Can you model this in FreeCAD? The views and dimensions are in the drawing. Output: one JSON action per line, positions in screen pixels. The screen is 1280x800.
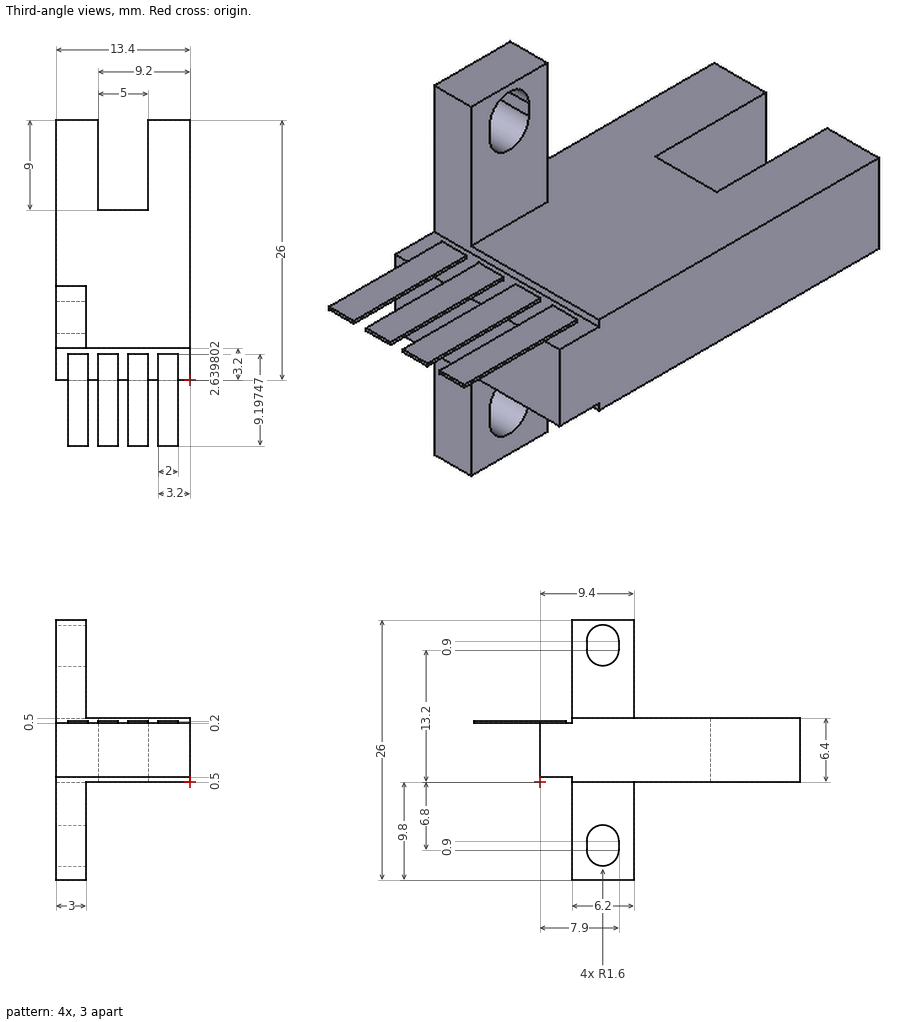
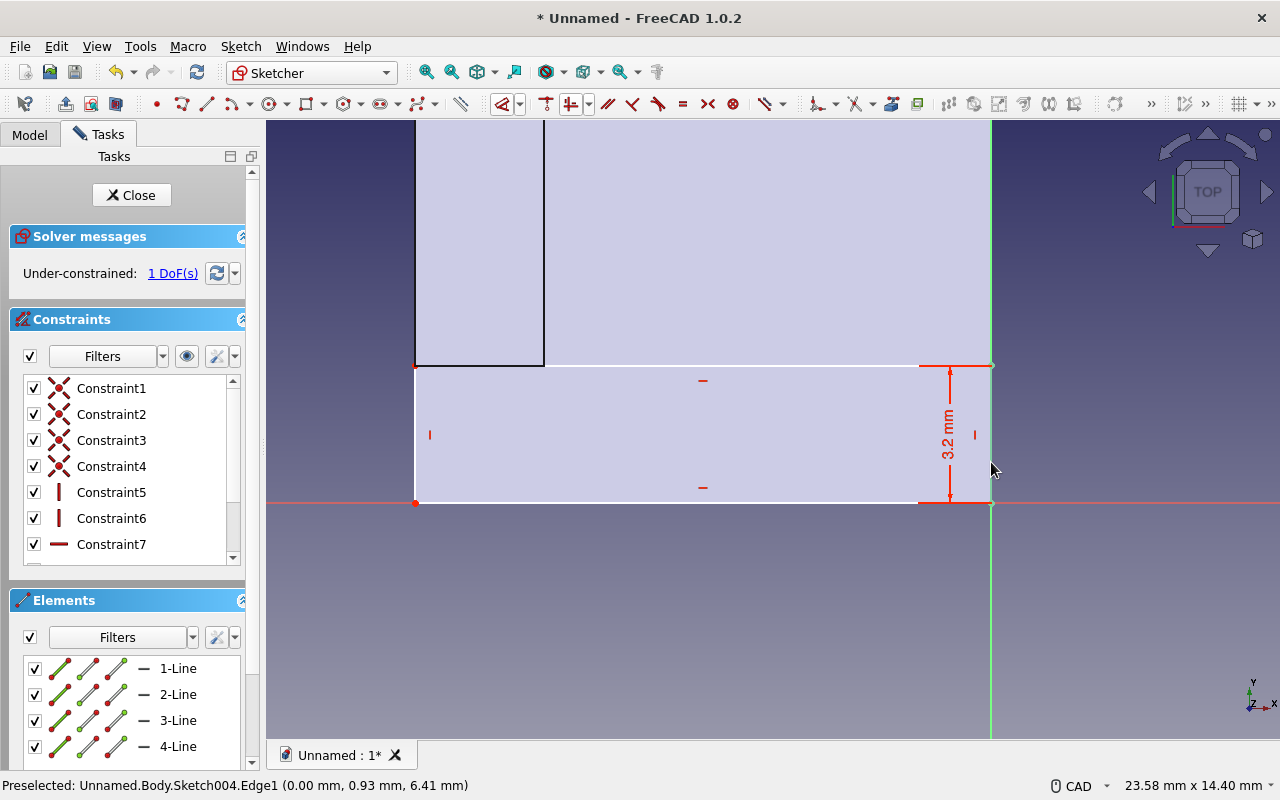
{"action": "left_click", "coordinate": [818, 366]}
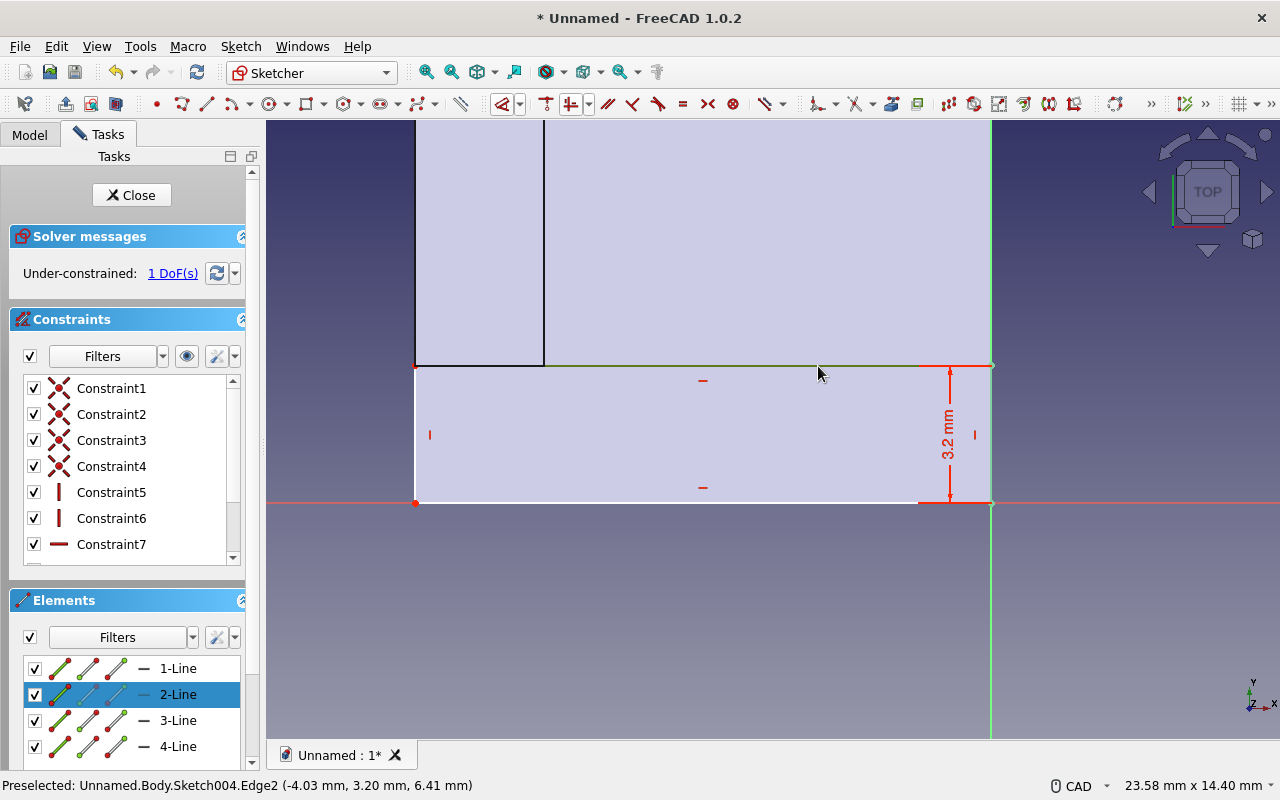
{"action": "key", "text": "l"}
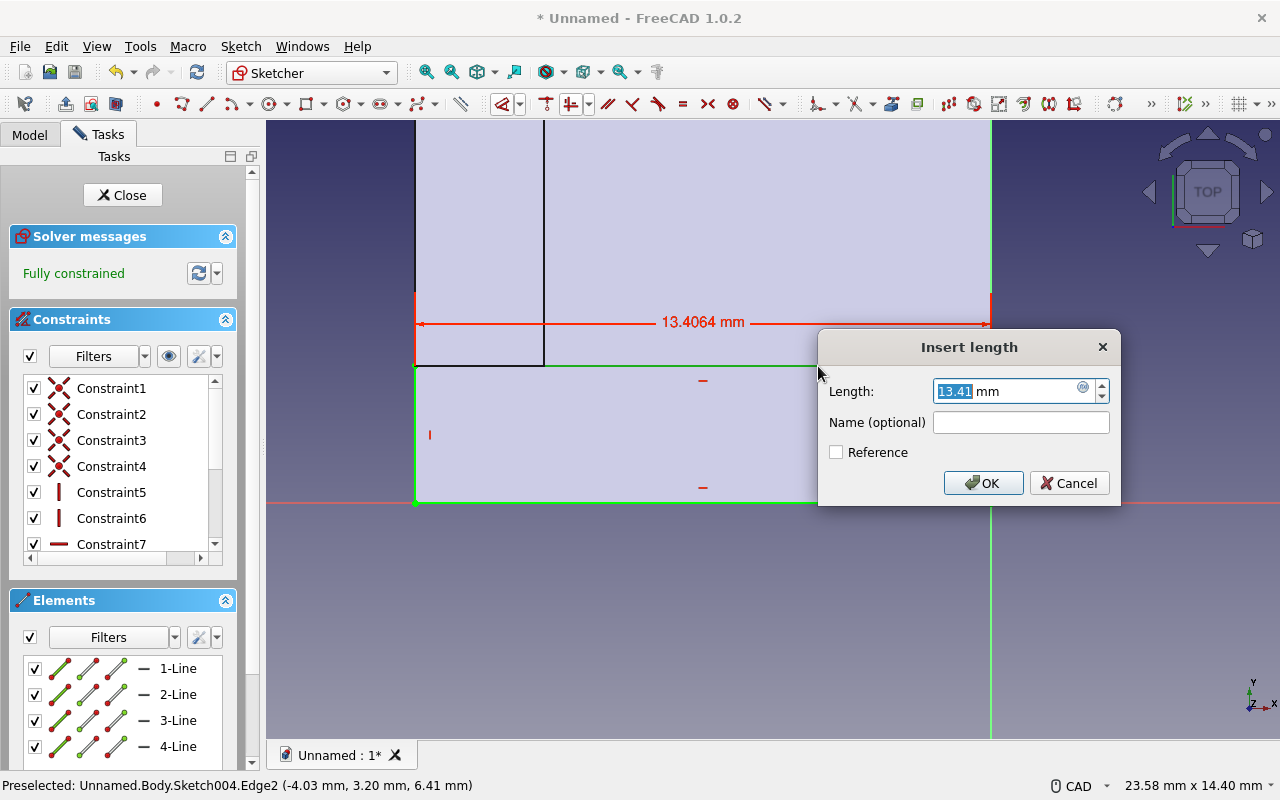
{"action": "type", "text": "13.4"}
{"action": "key", "text": "Return"}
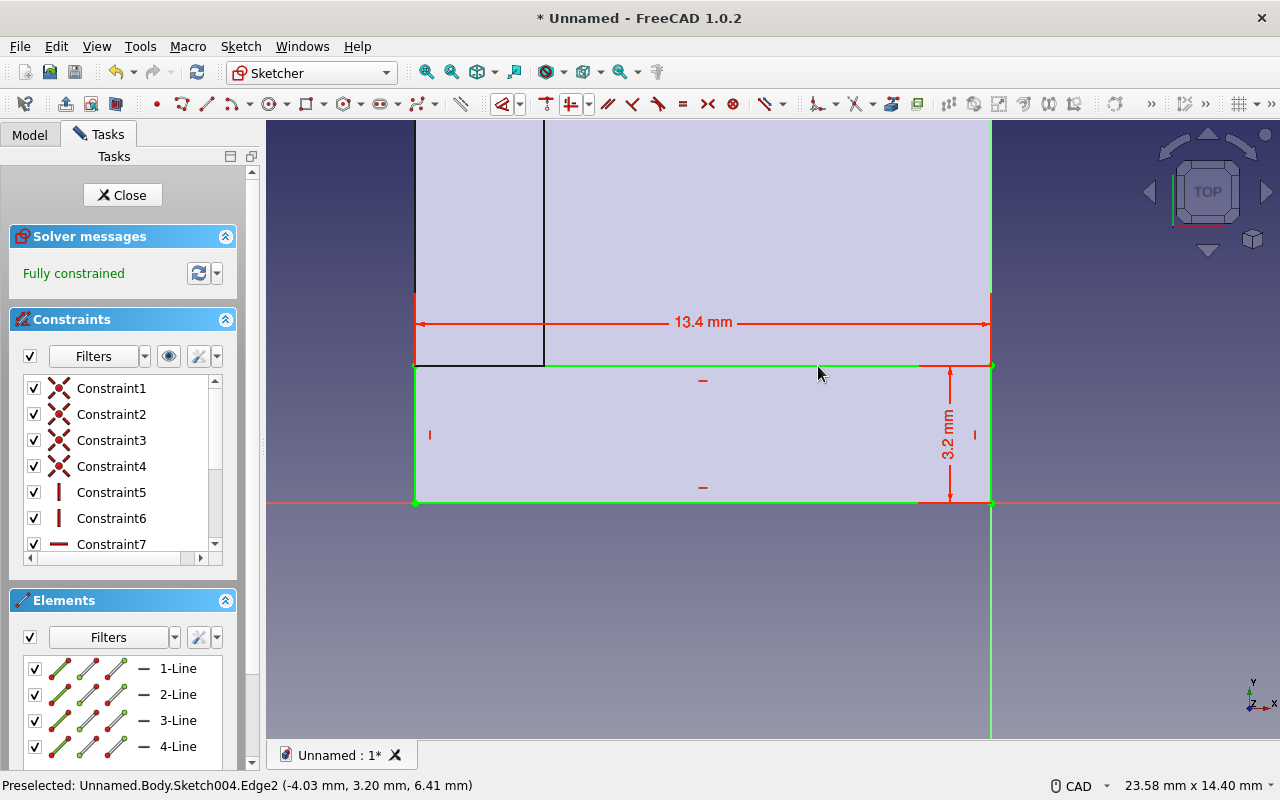
{"action": "left_click", "coordinate": [123, 195]}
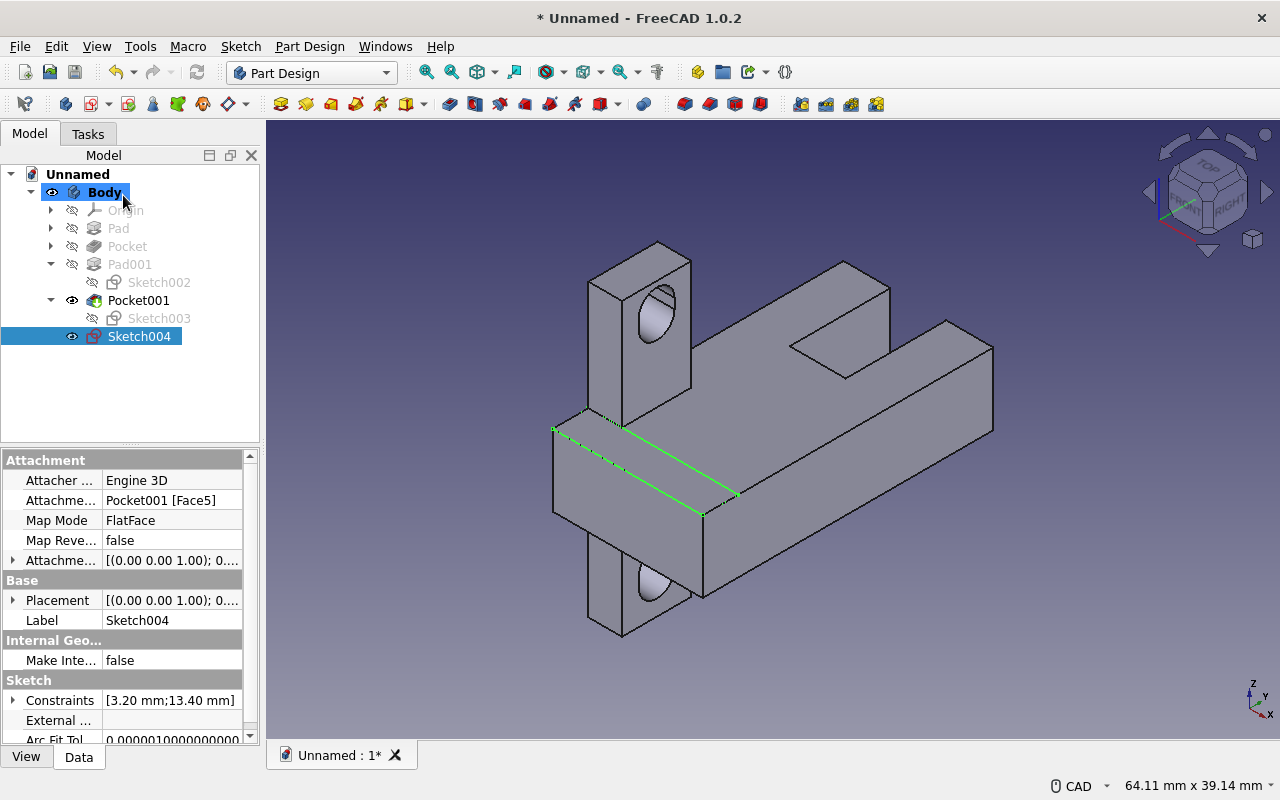
{"action": "left_click", "coordinate": [450, 104]}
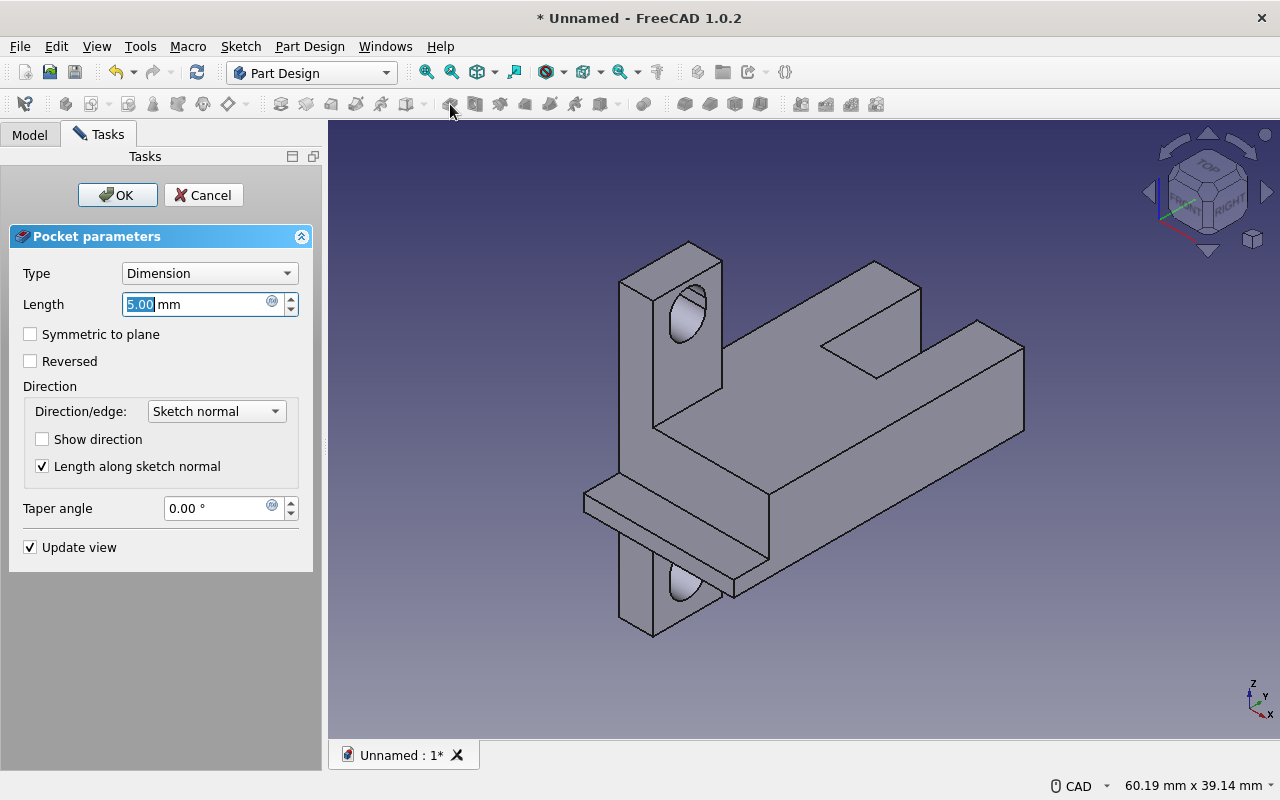
{"action": "type", "text": "0.5"}
{"action": "key", "text": "Tab"}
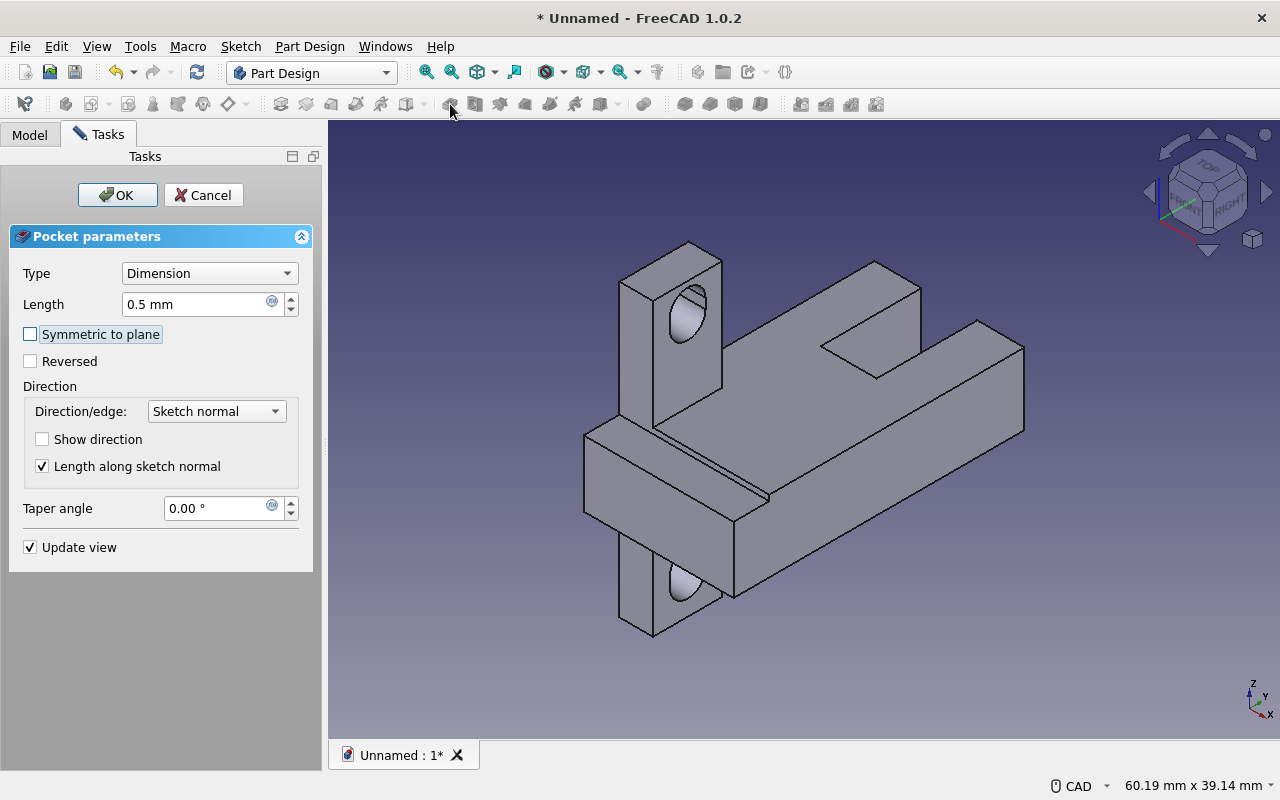
{"action": "left_click", "coordinate": [118, 195]}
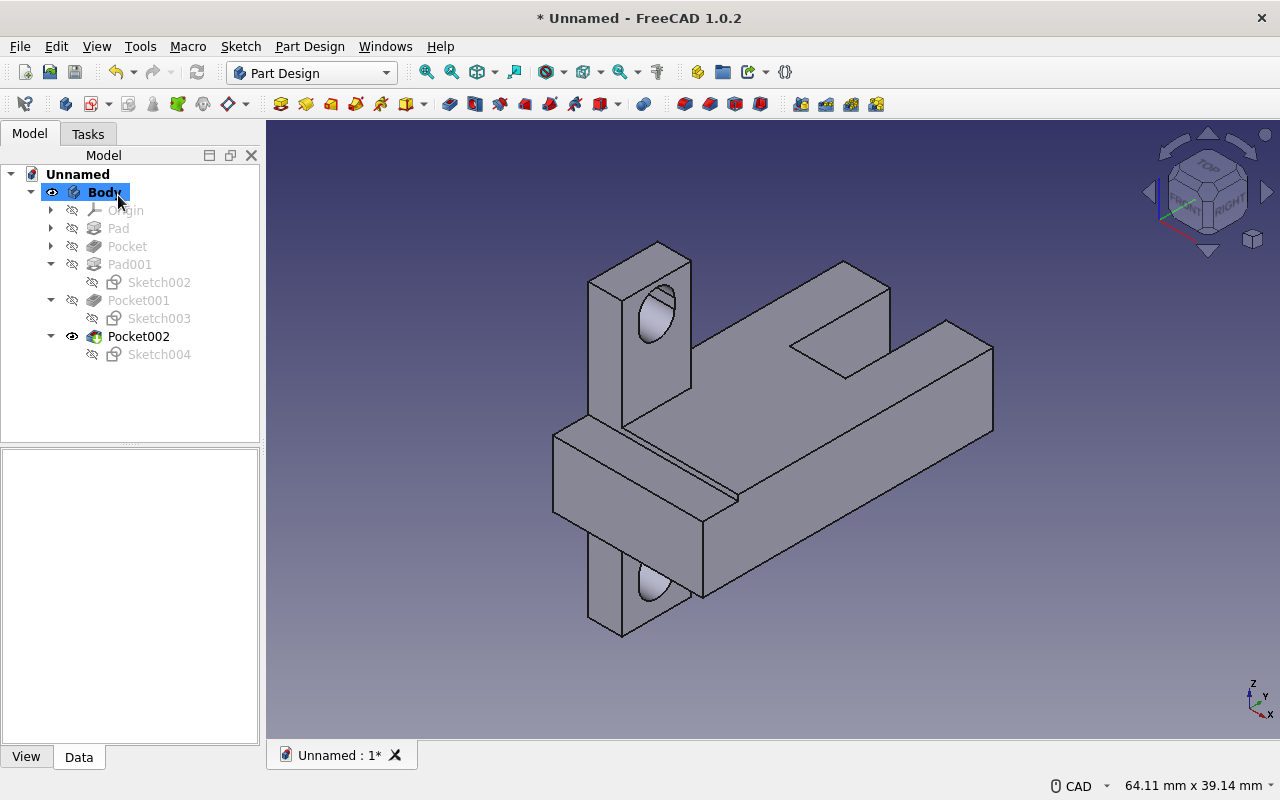
{"action": "left_click", "coordinate": [90, 104]}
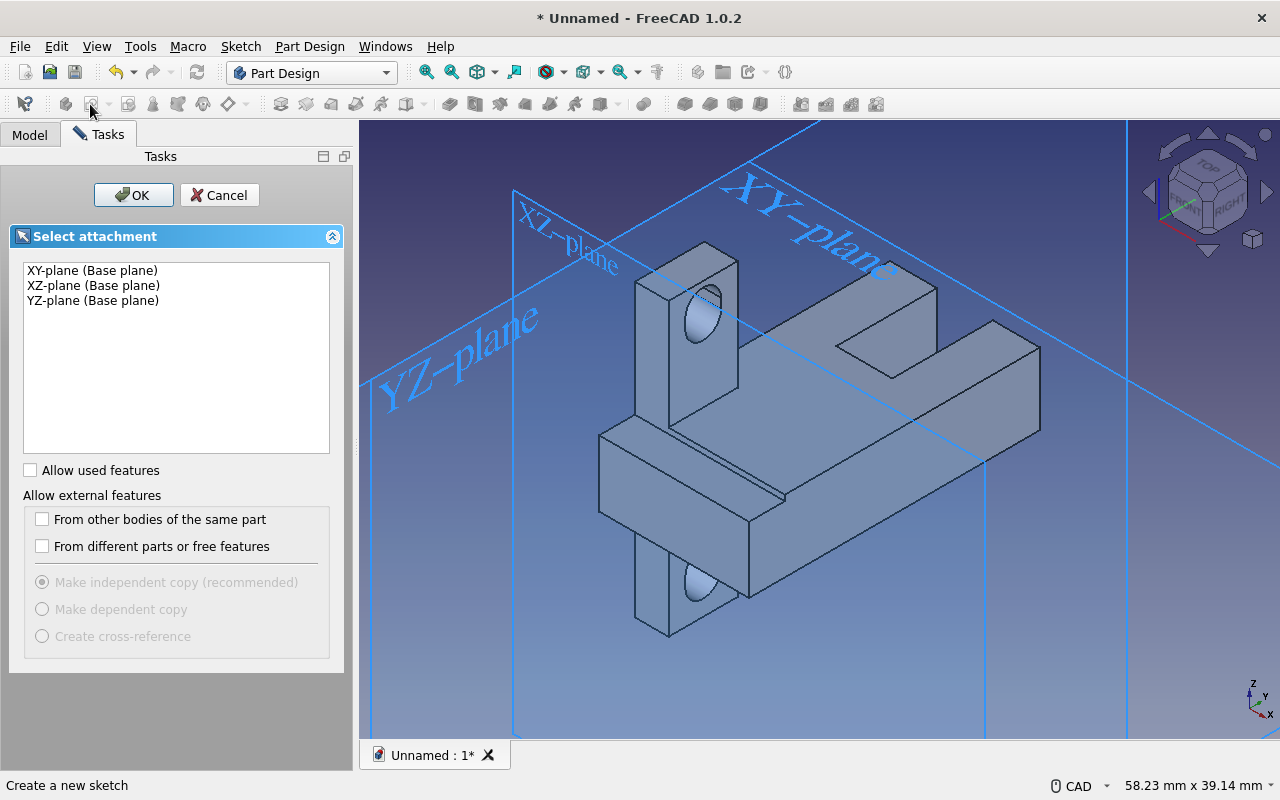
{"action": "left_click", "coordinate": [84, 270]}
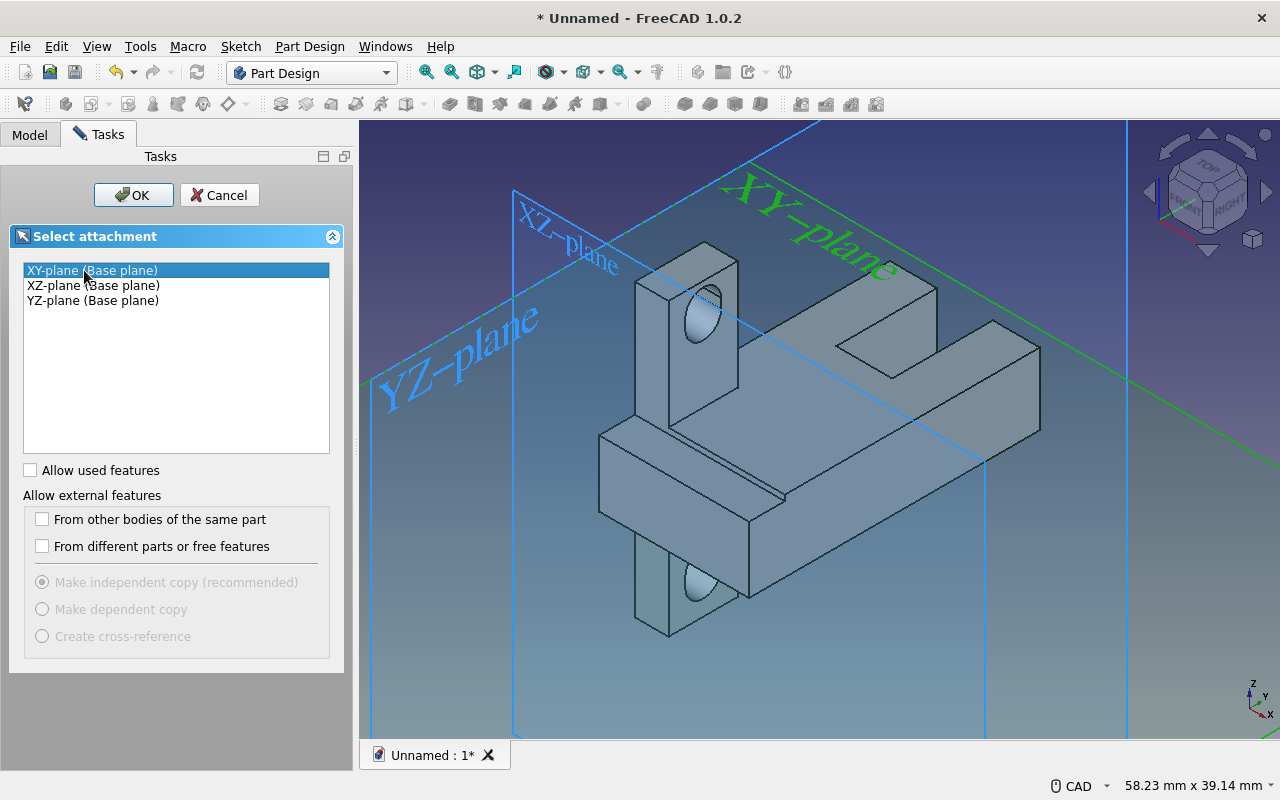
{"action": "left_click", "coordinate": [134, 195]}